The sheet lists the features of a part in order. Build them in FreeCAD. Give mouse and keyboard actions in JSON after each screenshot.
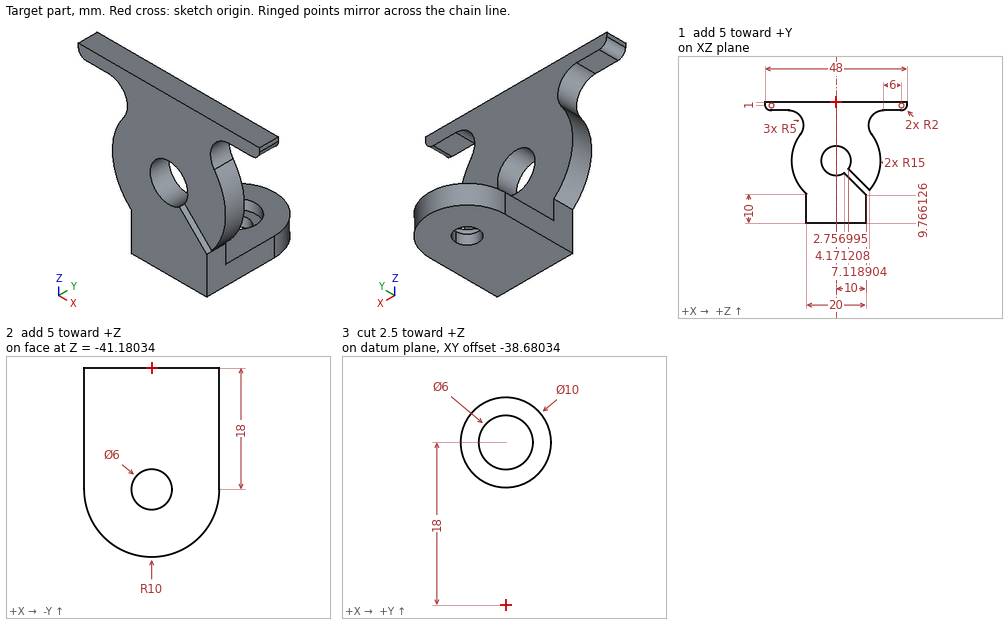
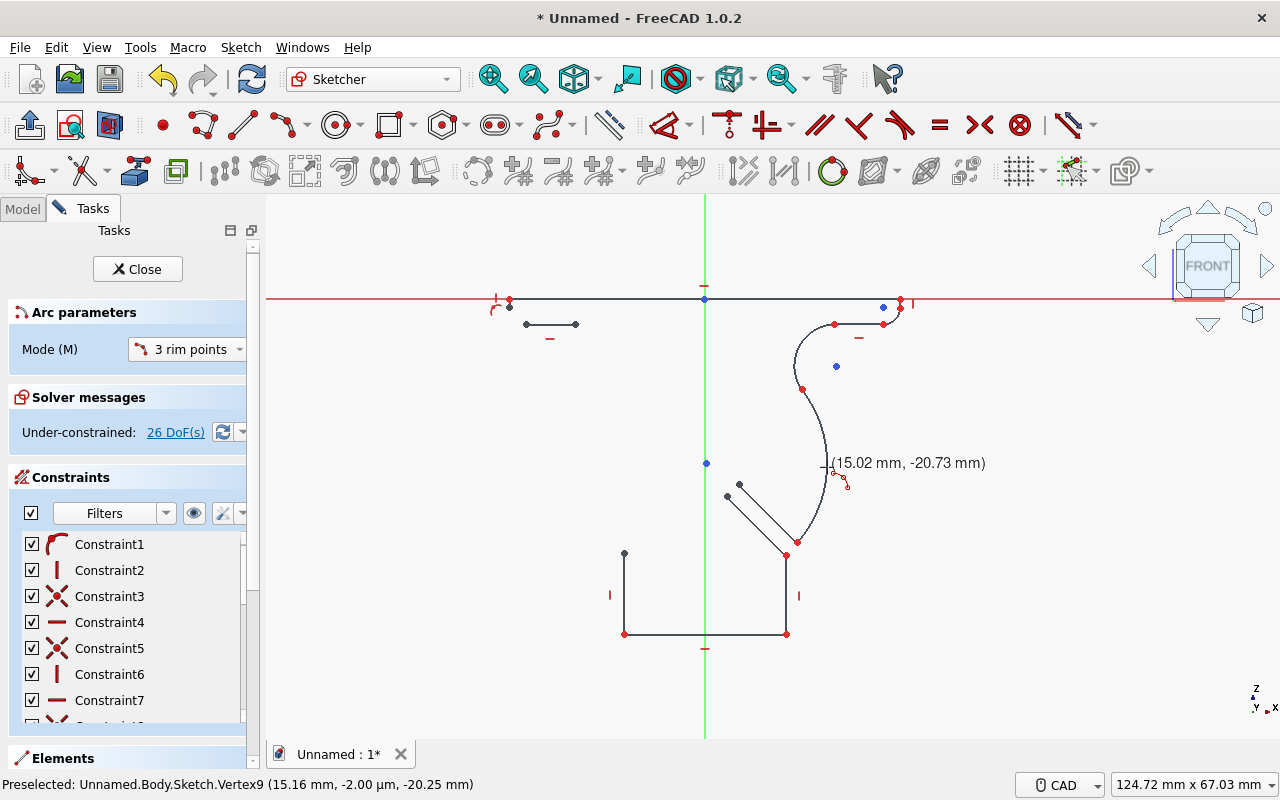
{"action": "left_click", "coordinate": [739, 485]}
{"action": "left_click", "coordinate": [727, 497]}
{"action": "left_click", "coordinate": [676, 433]}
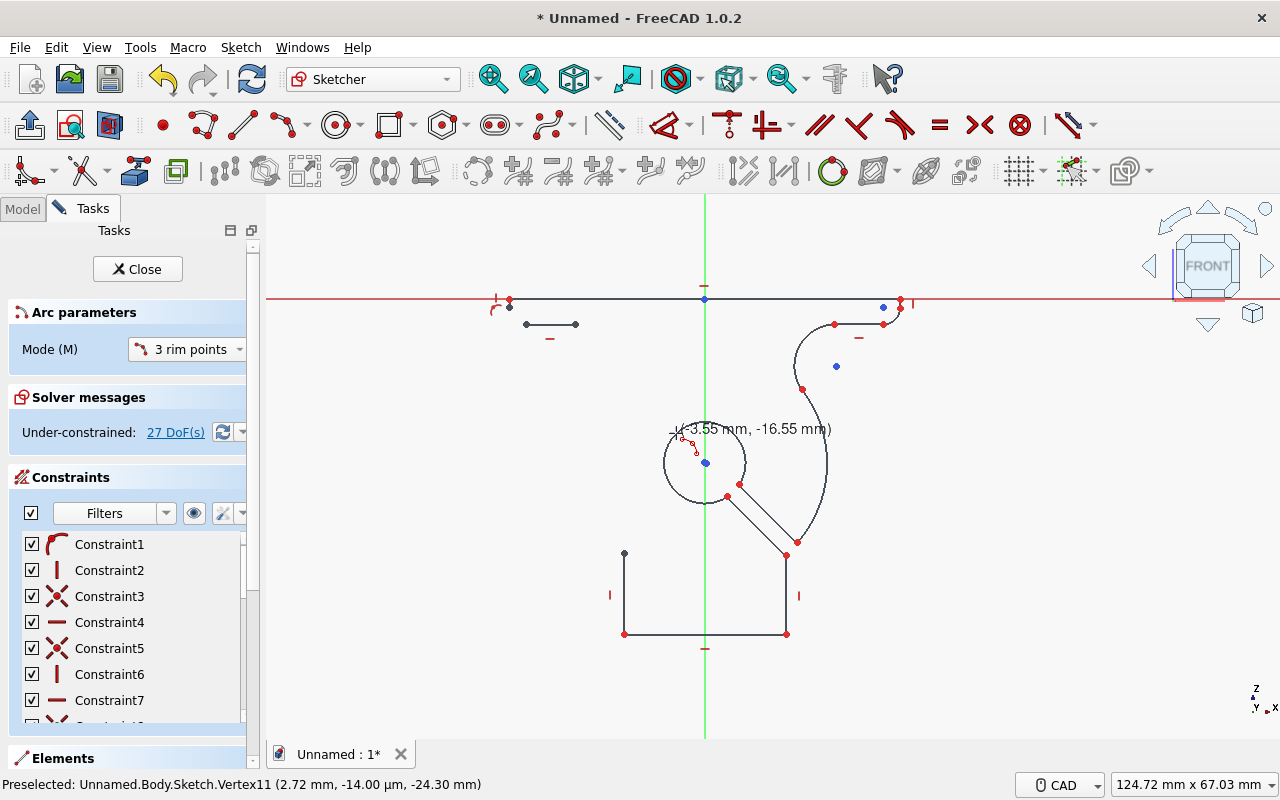
{"action": "left_click", "coordinate": [624, 554]}
{"action": "left_click", "coordinate": [607, 389]}
{"action": "left_click", "coordinate": [584, 474]}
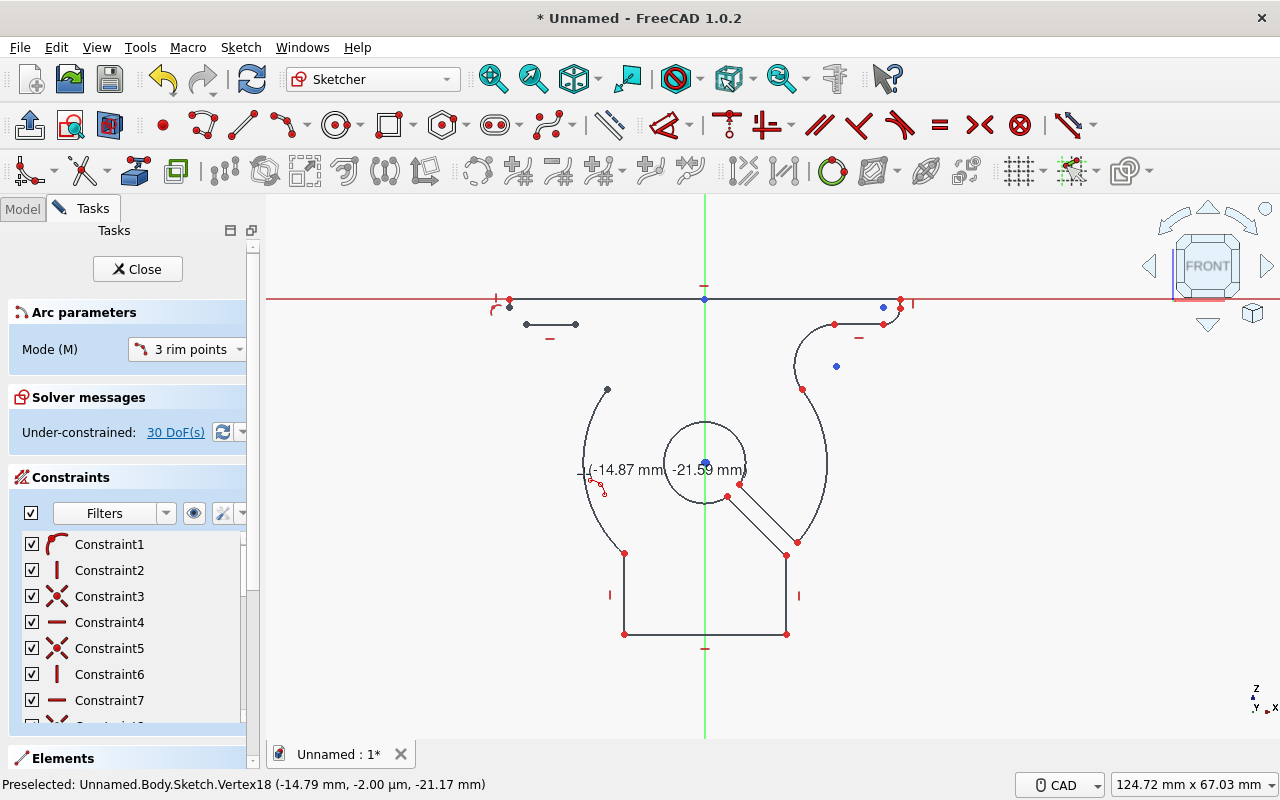
{"action": "left_click", "coordinate": [607, 390]}
{"action": "left_click", "coordinate": [575, 325]}
{"action": "left_click", "coordinate": [611, 346]}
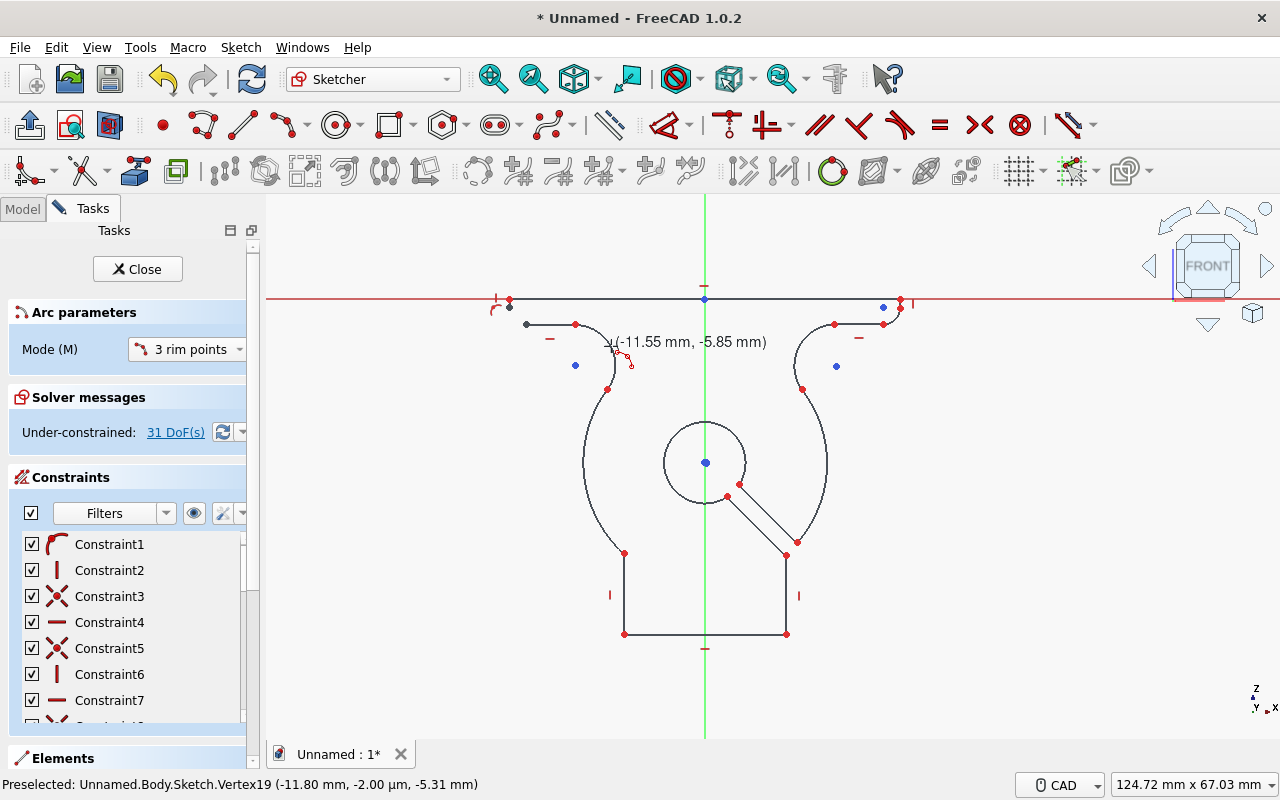
{"action": "left_click", "coordinate": [526, 325]}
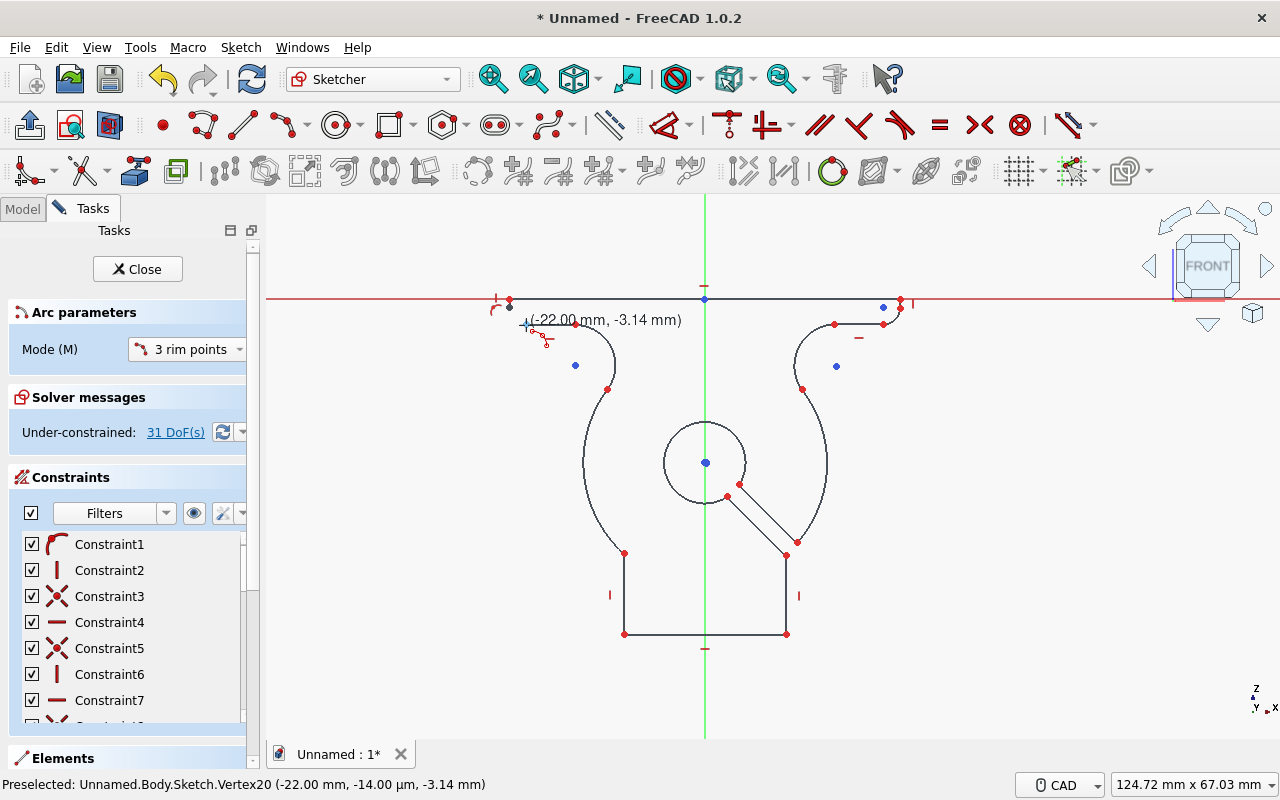
{"action": "scroll", "coordinate": [510, 308], "scroll_direction": "up", "scroll_amount": 7}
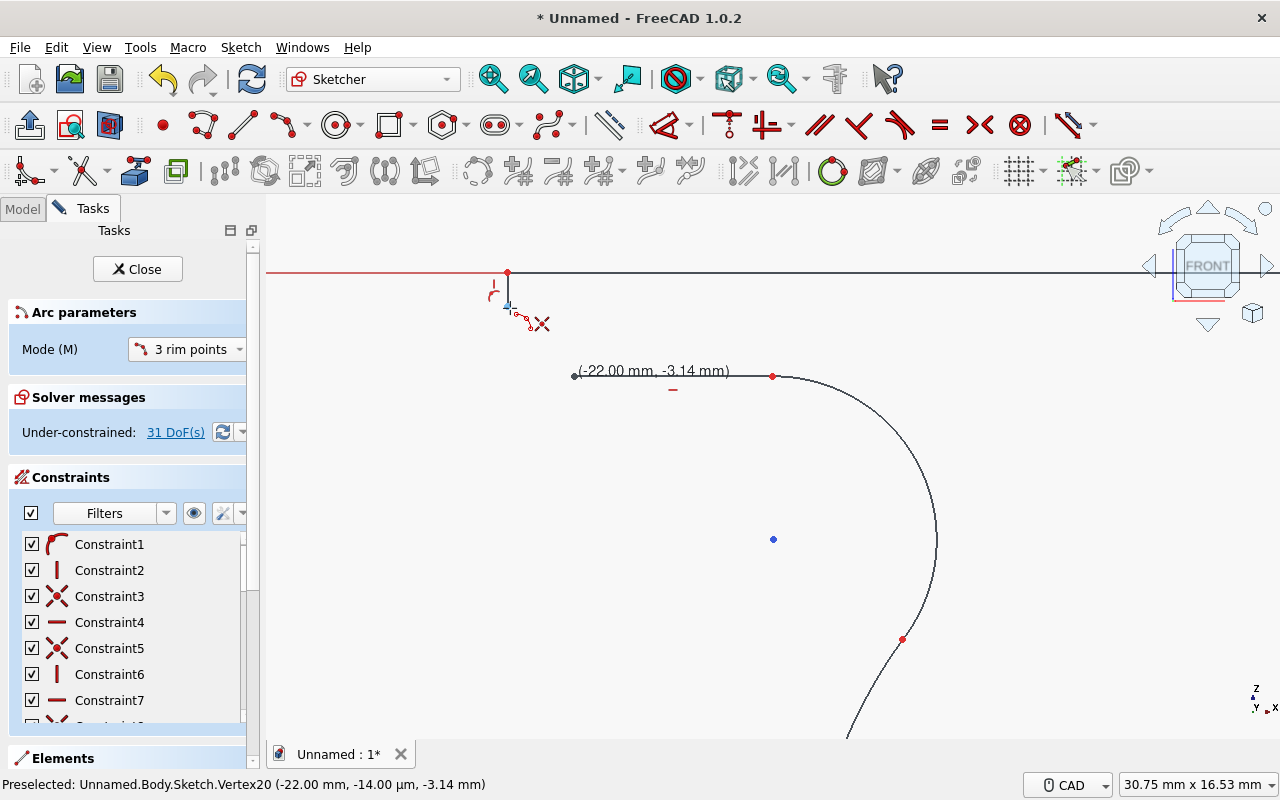
{"action": "left_click", "coordinate": [508, 307]}
{"action": "left_click", "coordinate": [528, 352]}
{"action": "key", "text": "Escape"}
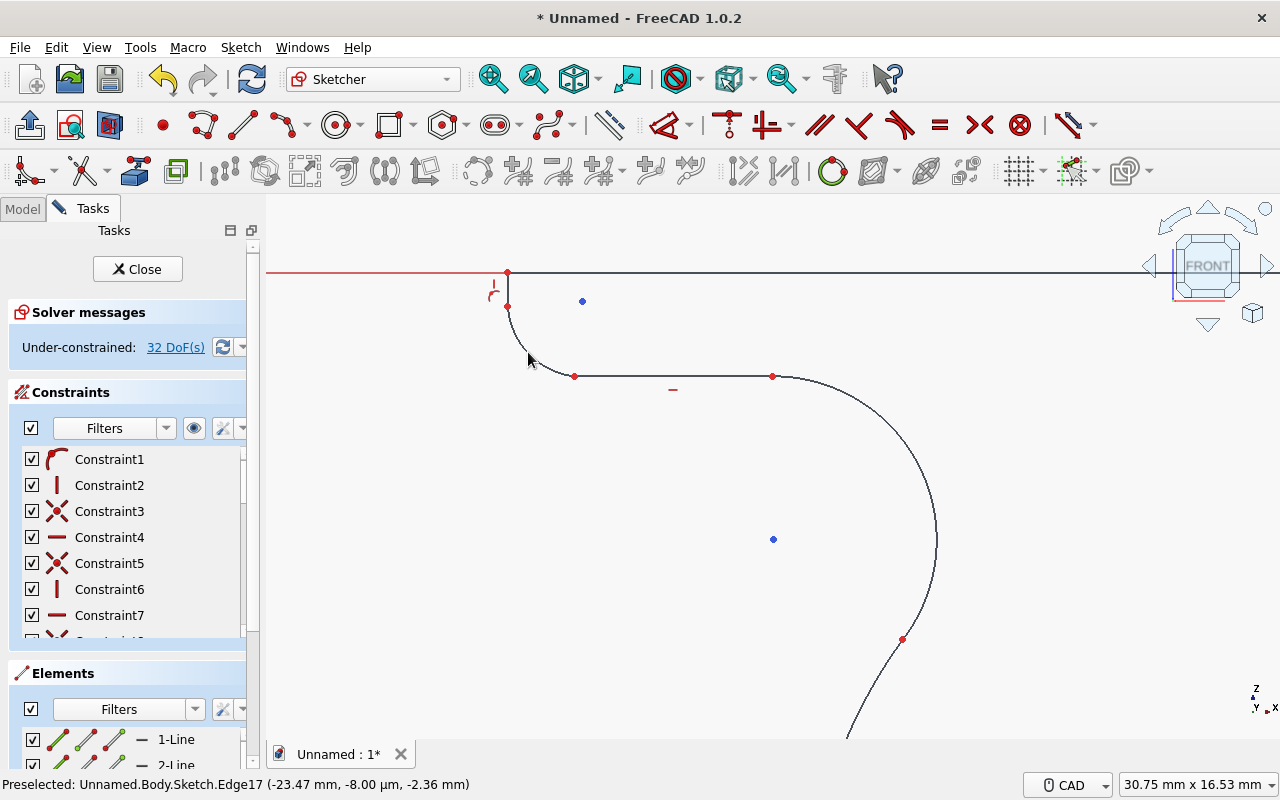
{"action": "scroll", "coordinate": [508, 296], "scroll_direction": "up", "scroll_amount": 2}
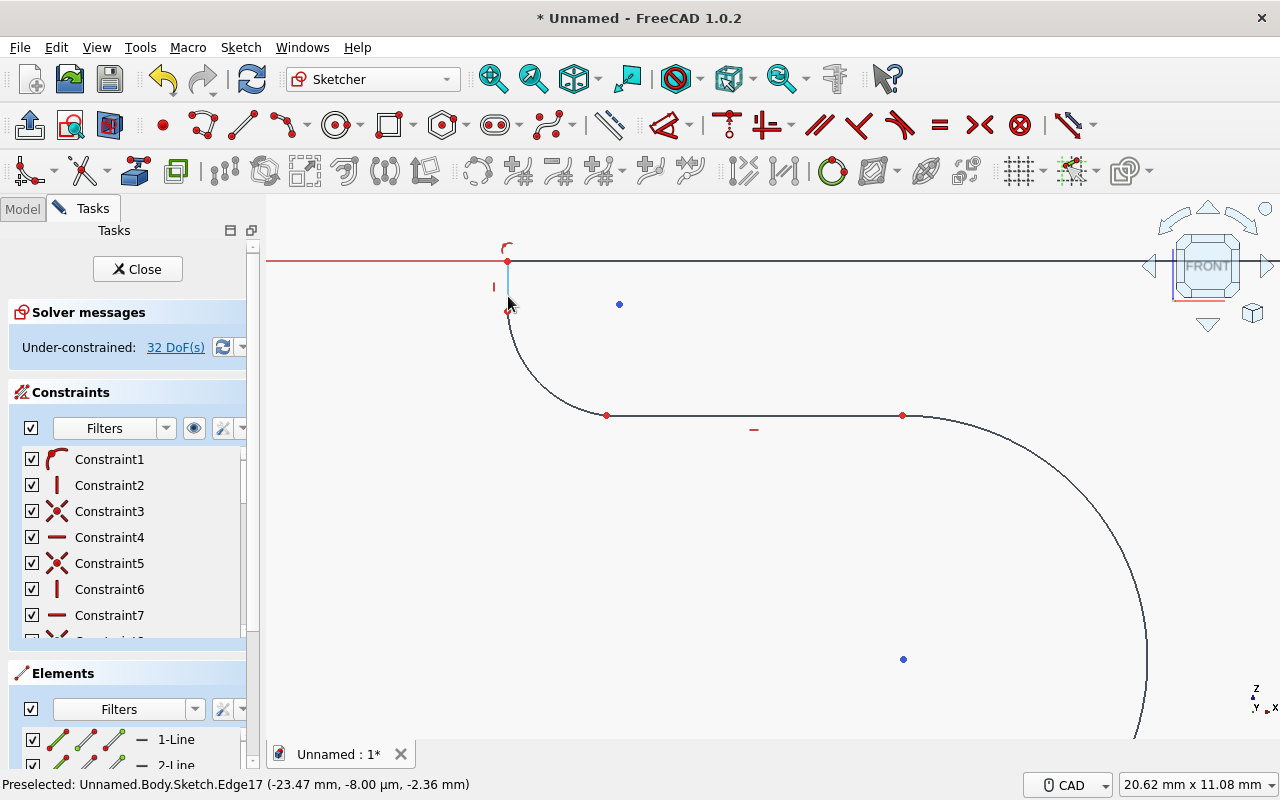
{"action": "left_click", "coordinate": [508, 297]}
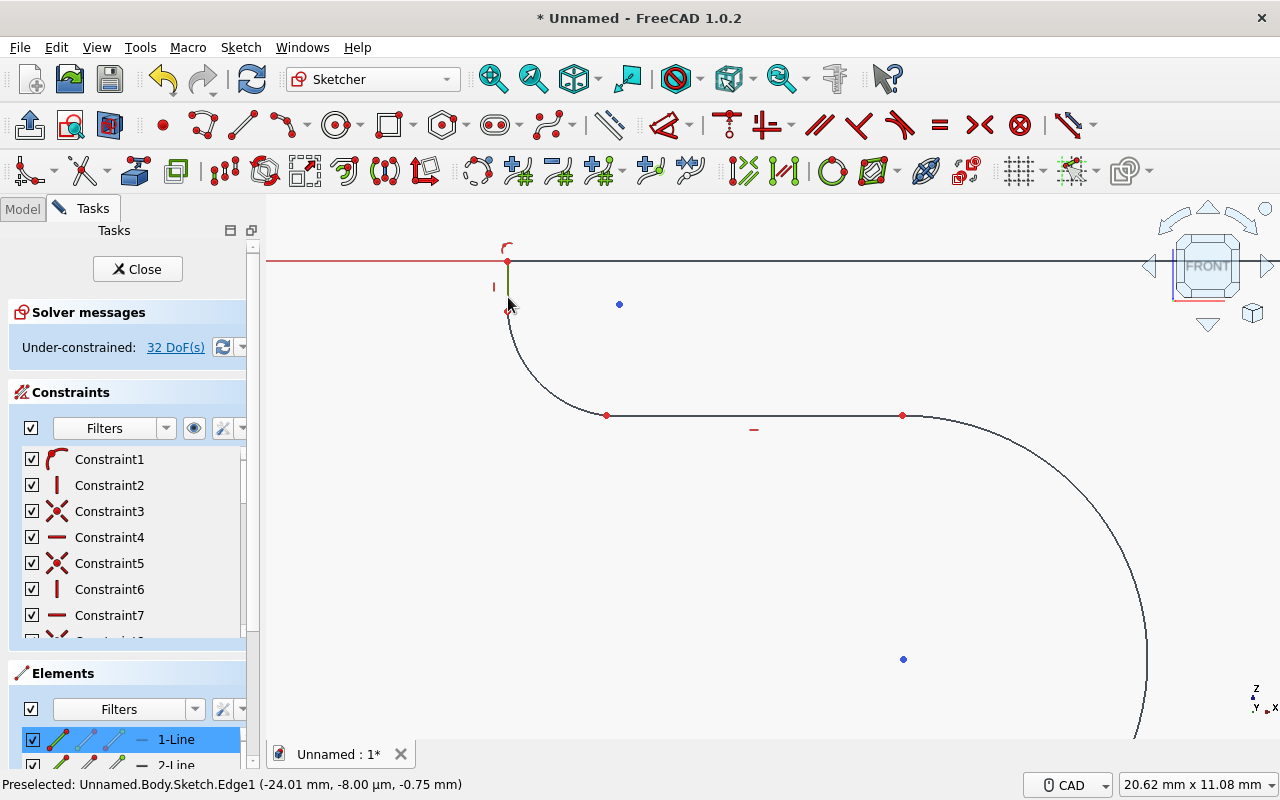
{"action": "scroll", "coordinate": [510, 307], "scroll_direction": "down", "scroll_amount": 9}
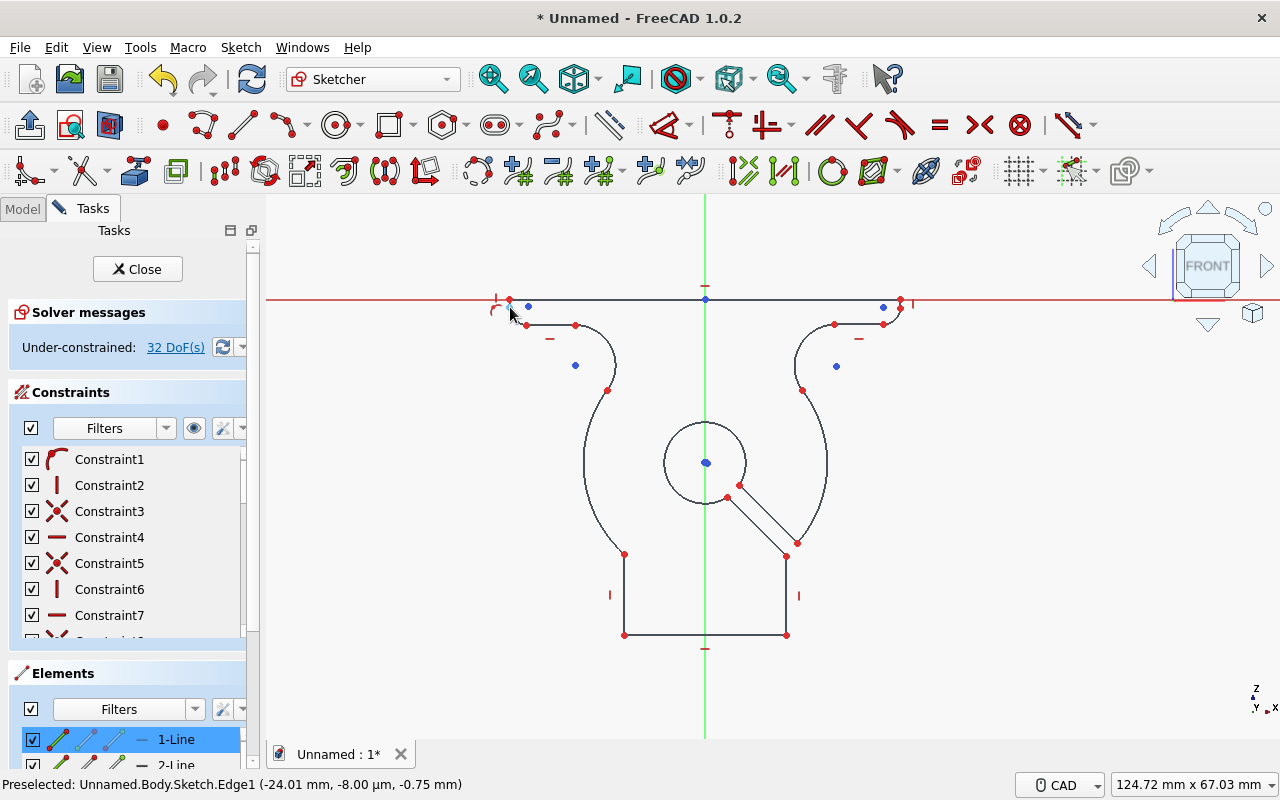
{"action": "scroll", "coordinate": [512, 315], "scroll_direction": "up", "scroll_amount": 3}